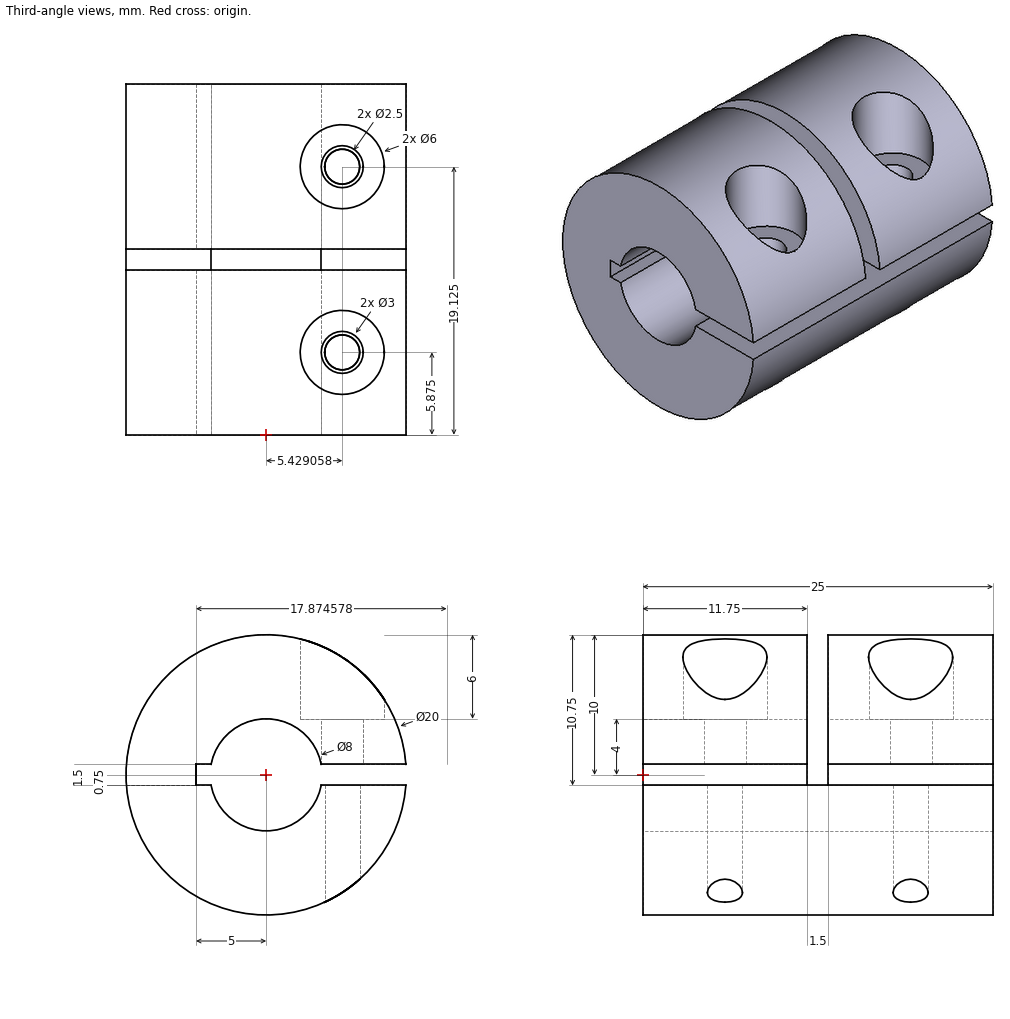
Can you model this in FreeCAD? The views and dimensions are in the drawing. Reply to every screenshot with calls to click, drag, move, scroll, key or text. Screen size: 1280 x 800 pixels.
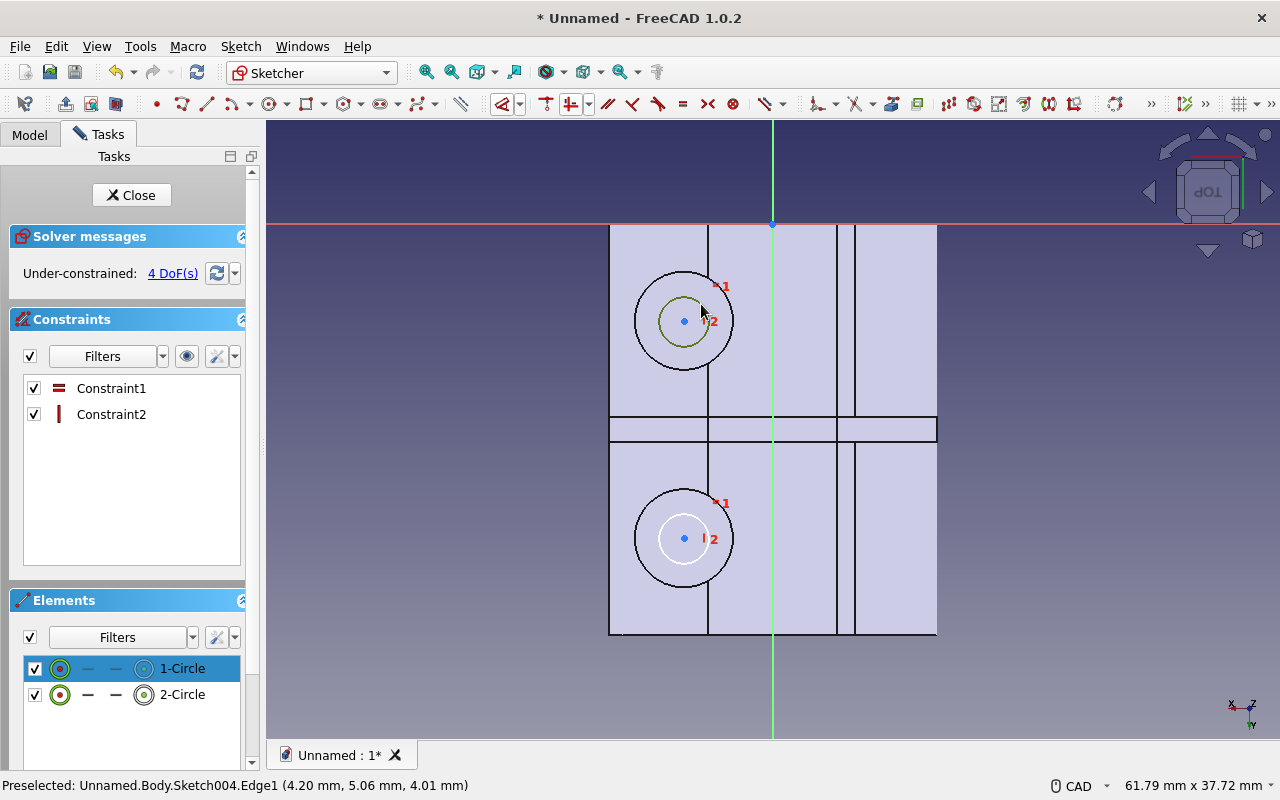
click(520, 104)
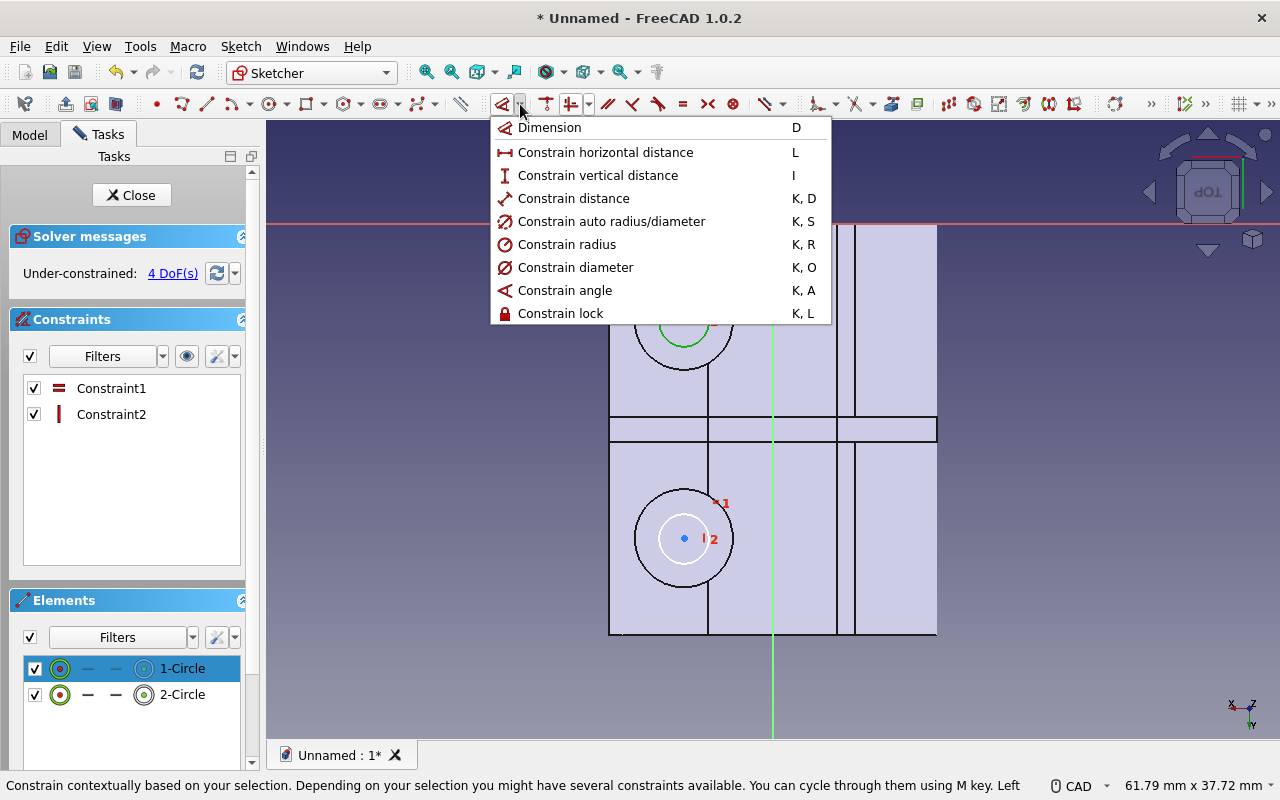
click(661, 268)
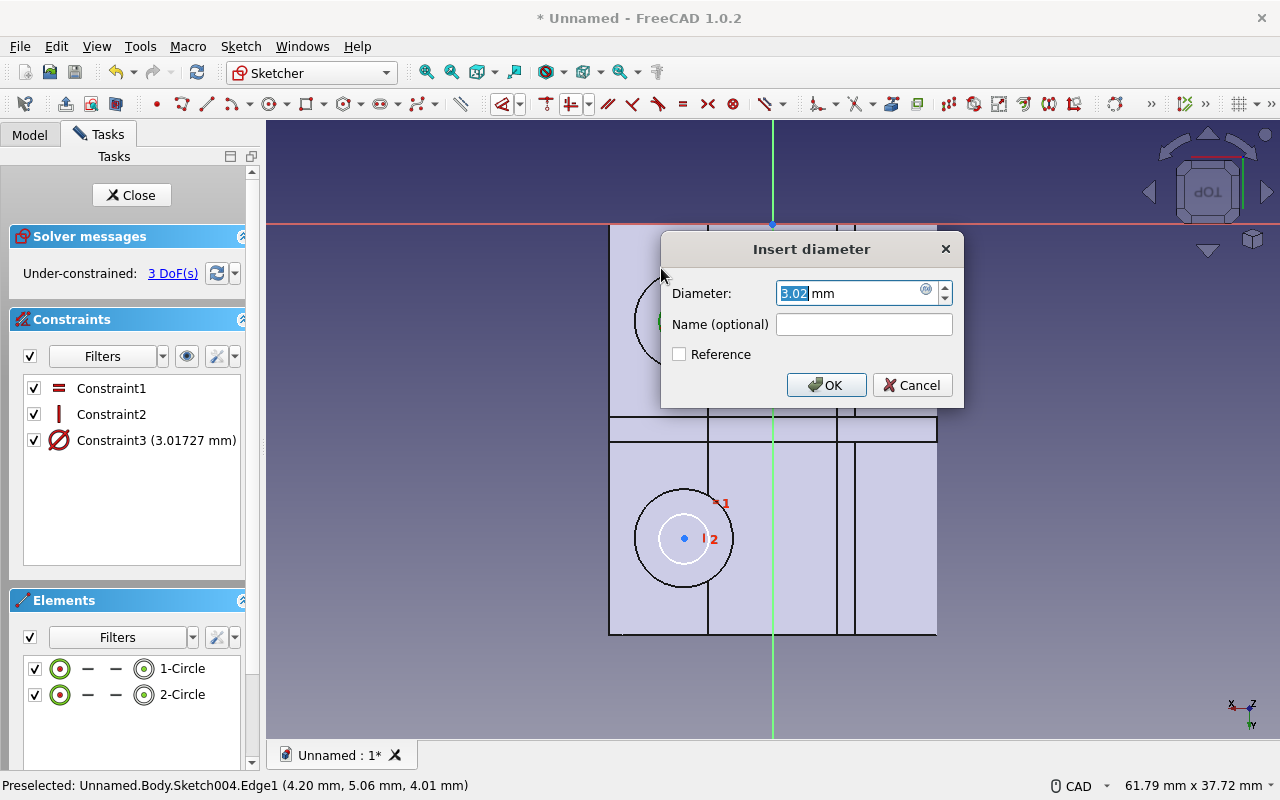
text(3)
key(Return)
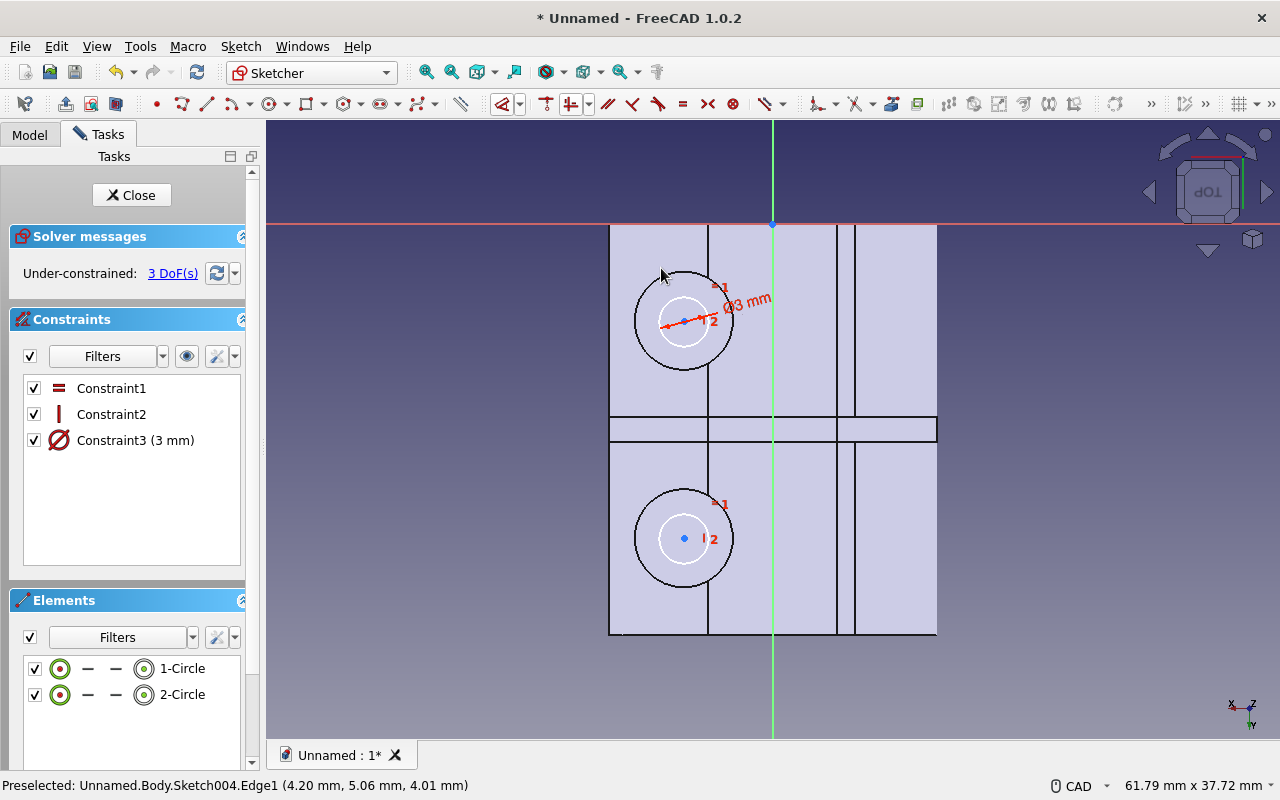
click(684, 322)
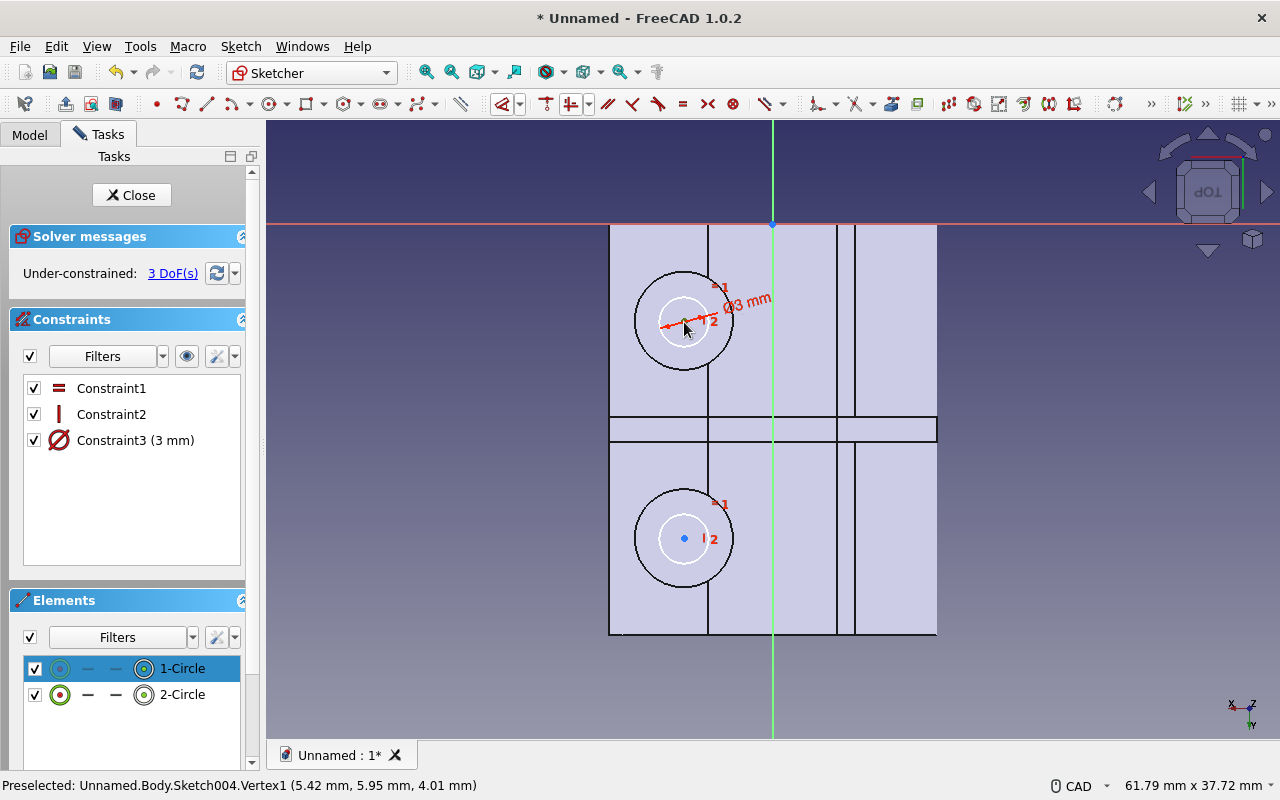
click(520, 104)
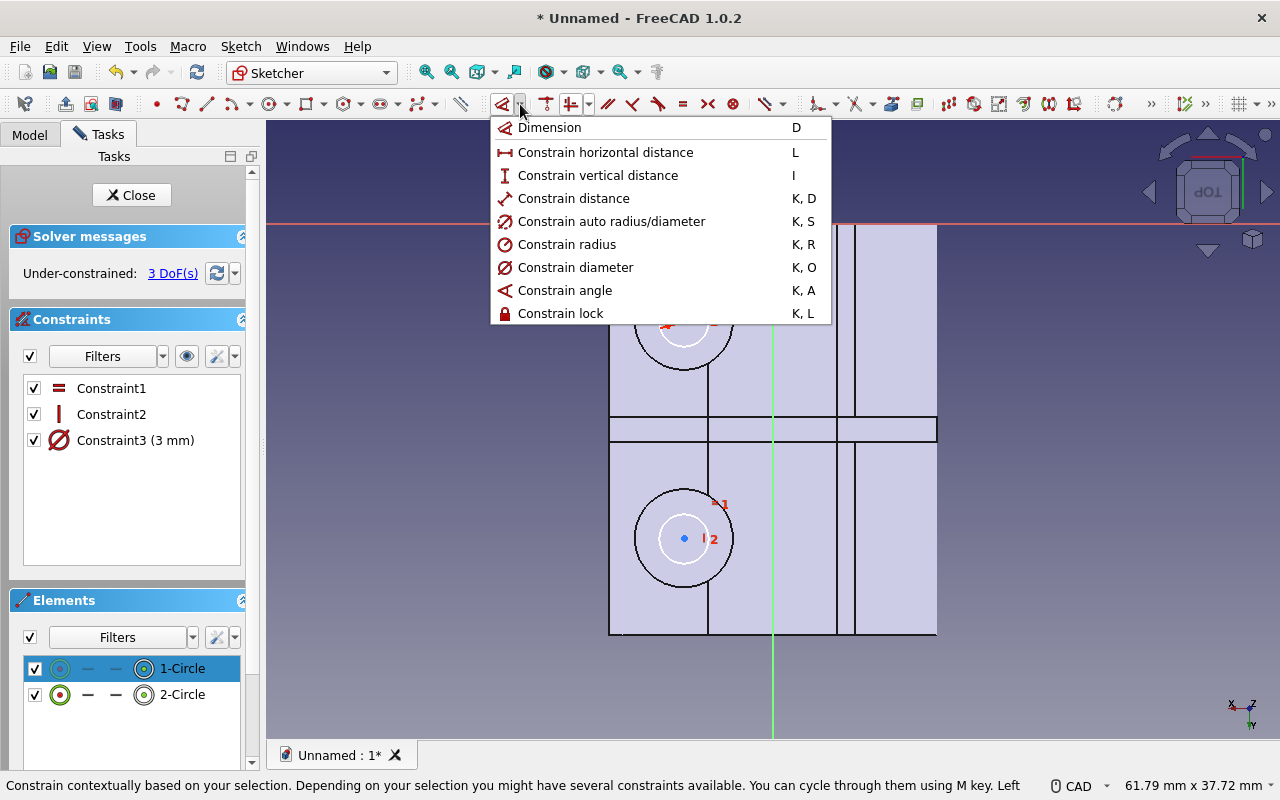
click(661, 176)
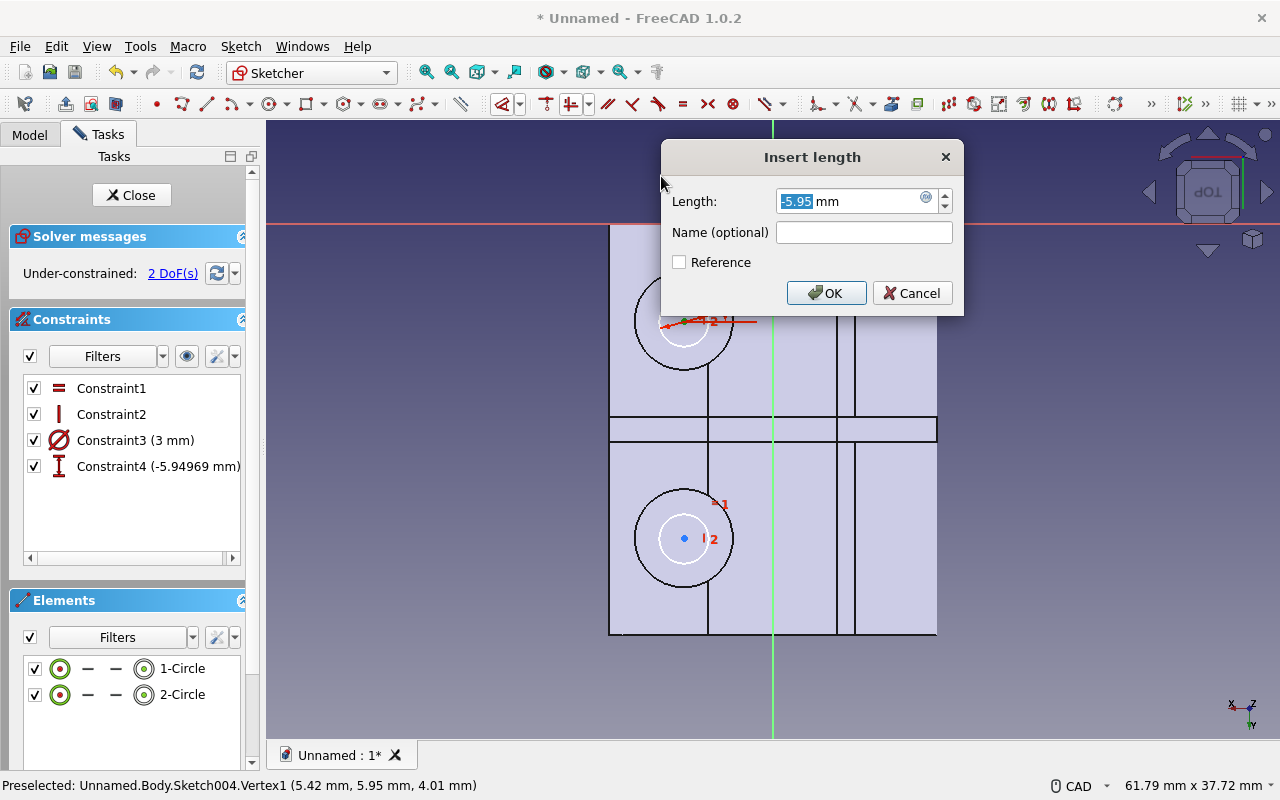
text(-5.875)
key(Return)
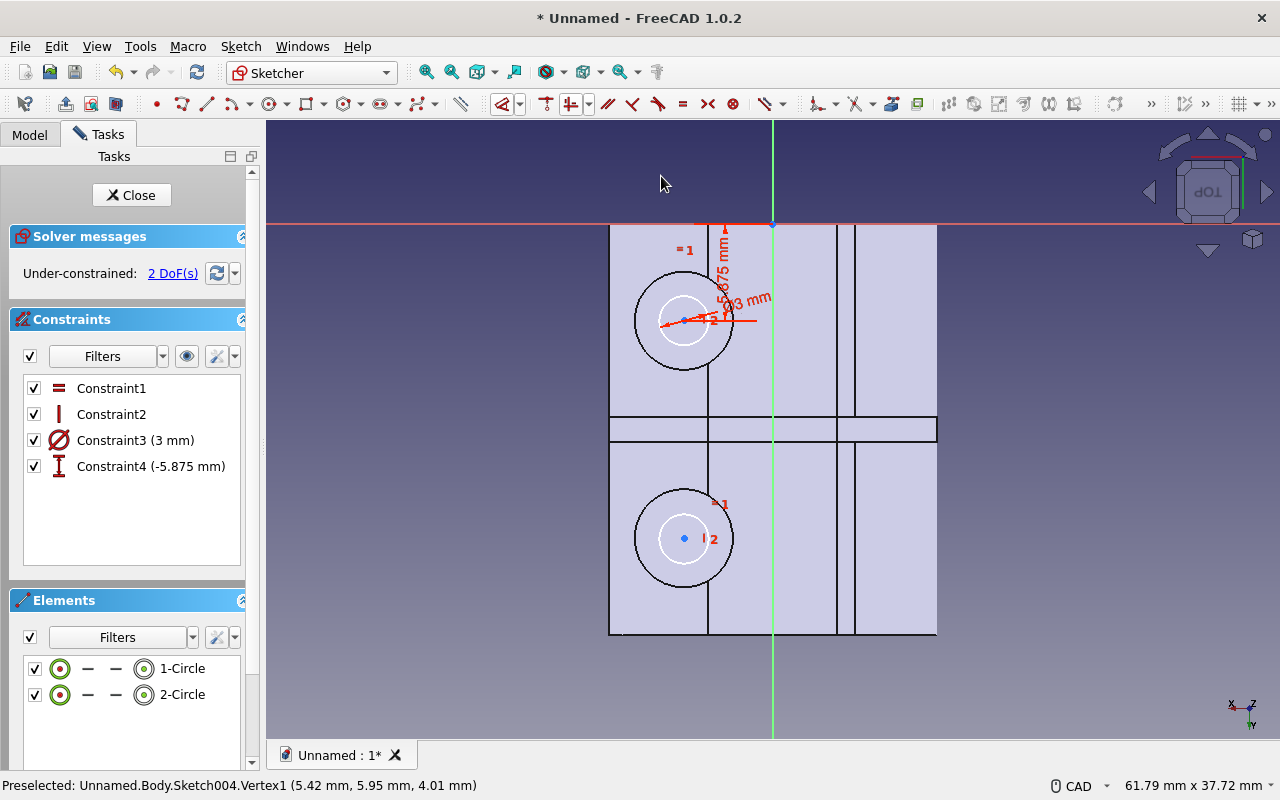
click(684, 539)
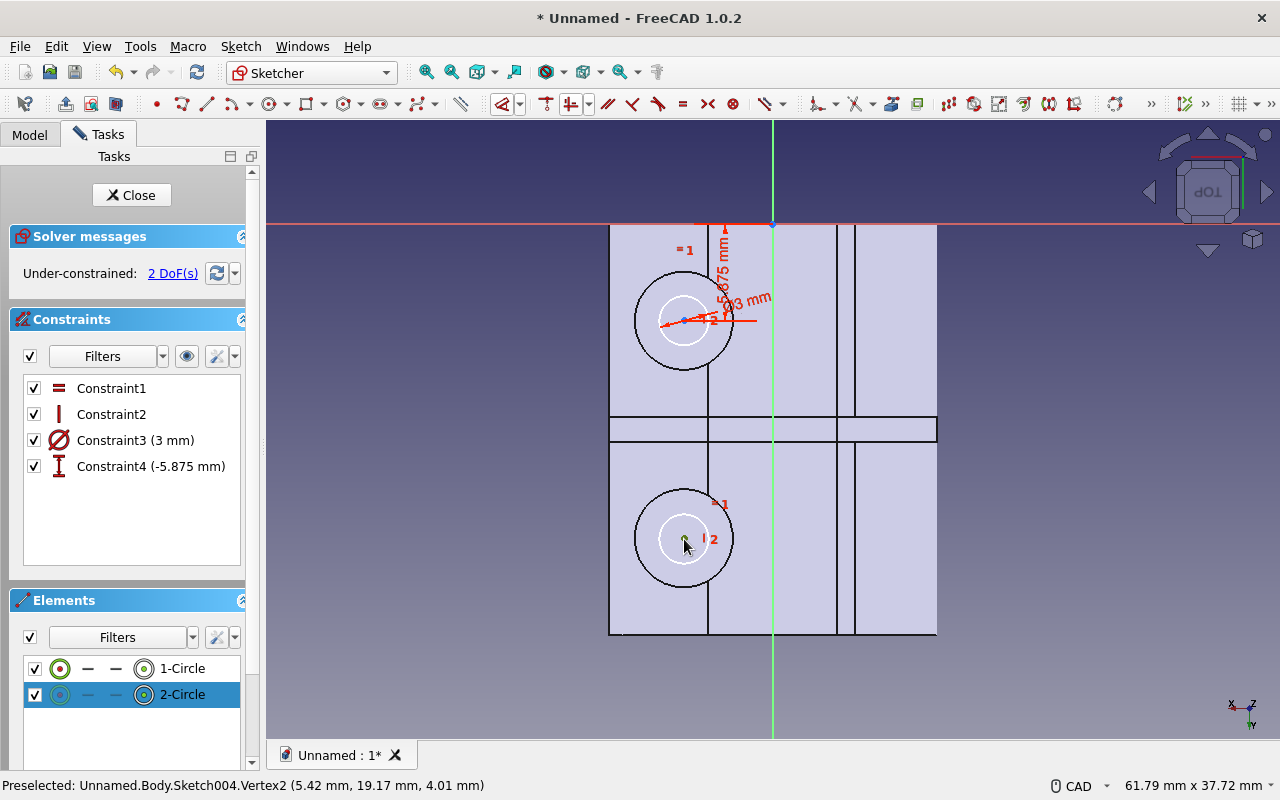
key(i)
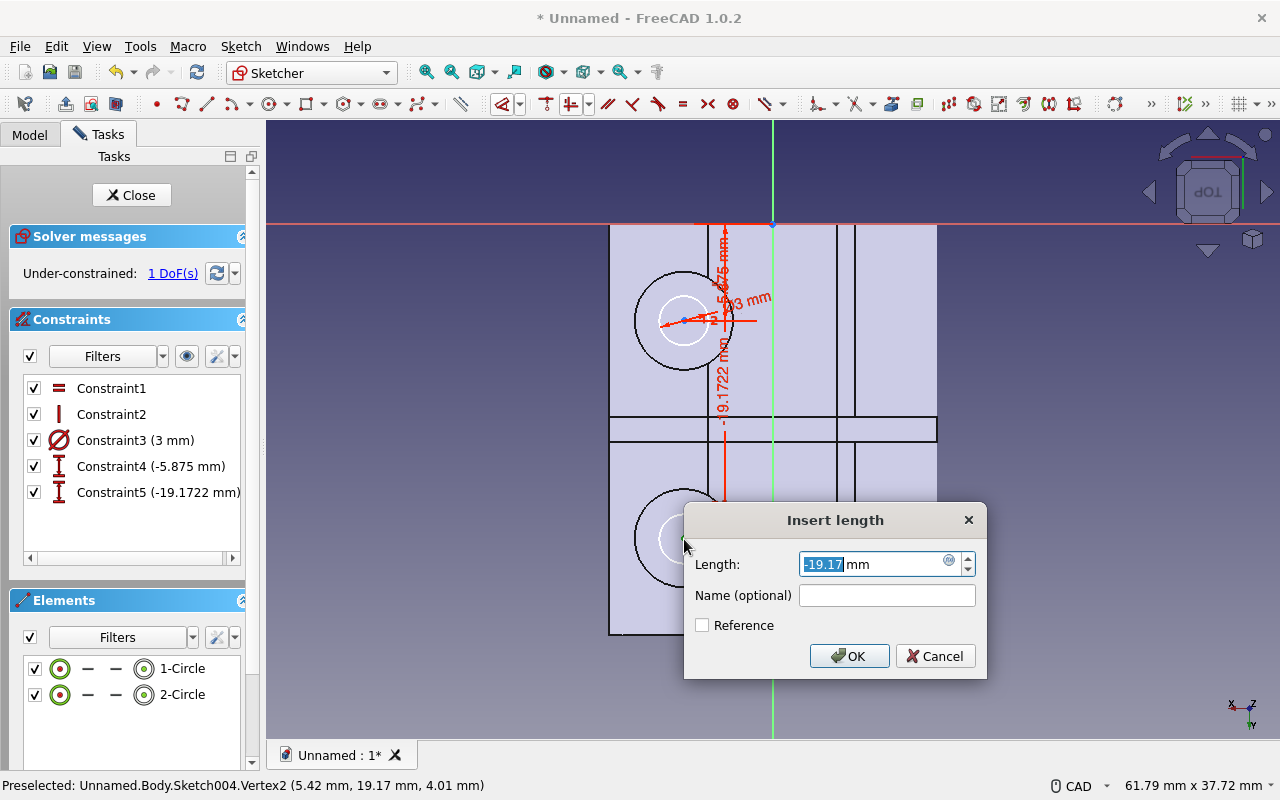
text(-19.125)
key(Return)